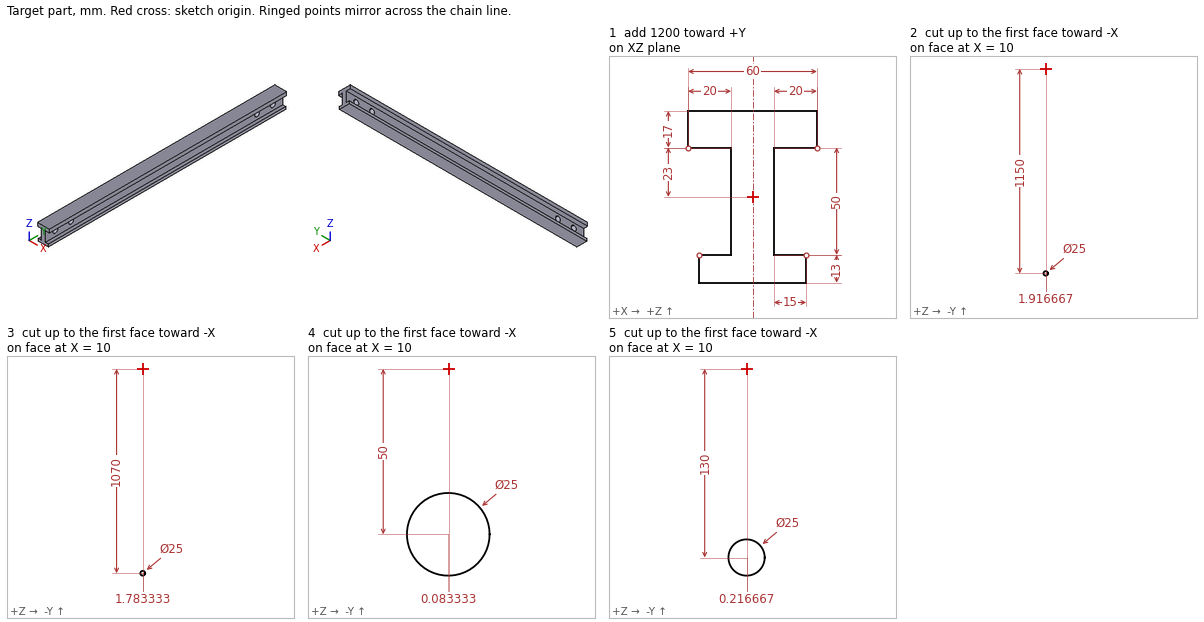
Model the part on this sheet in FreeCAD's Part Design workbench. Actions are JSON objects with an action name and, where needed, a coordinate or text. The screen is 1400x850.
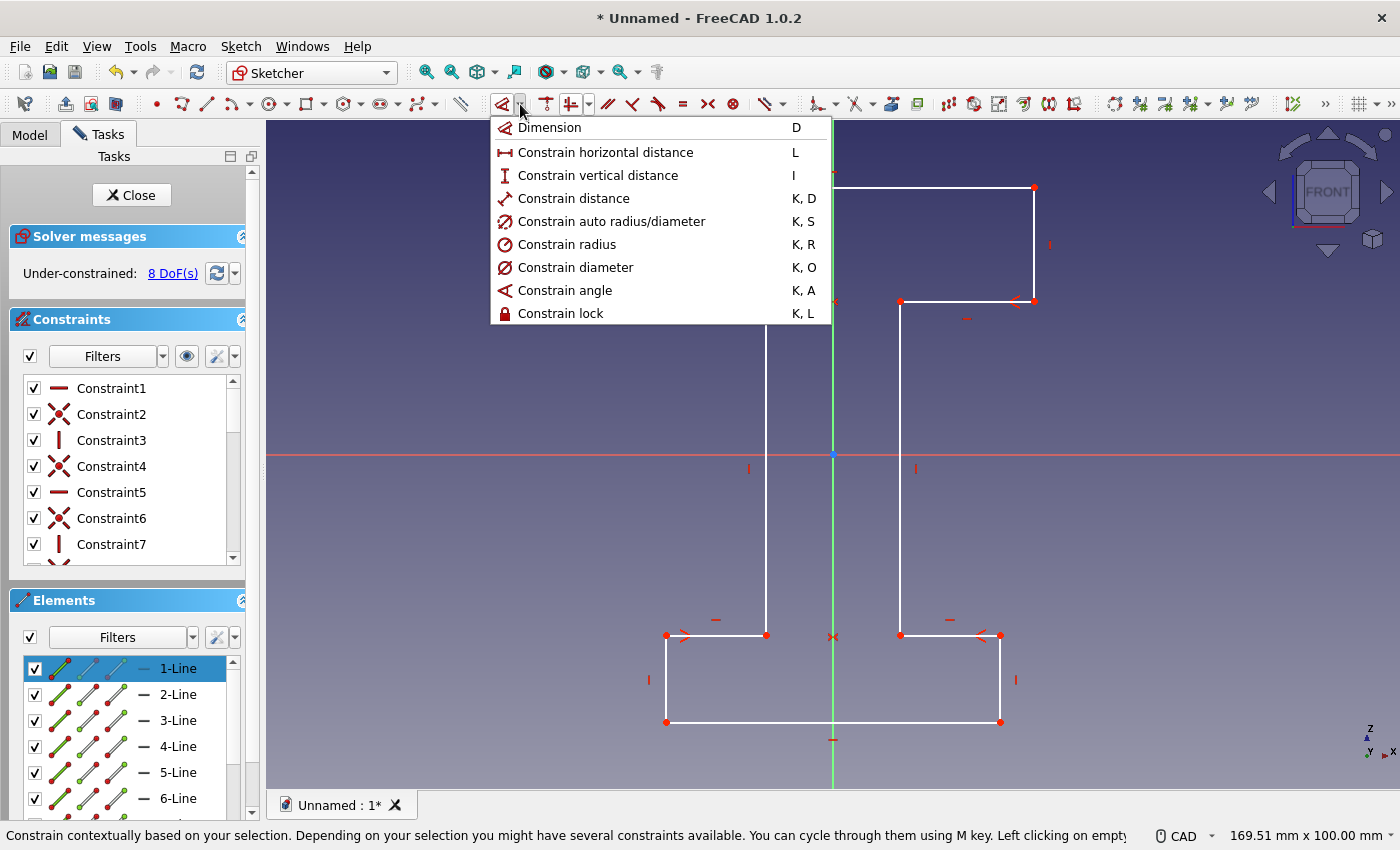
{"action": "left_click", "coordinate": [661, 152]}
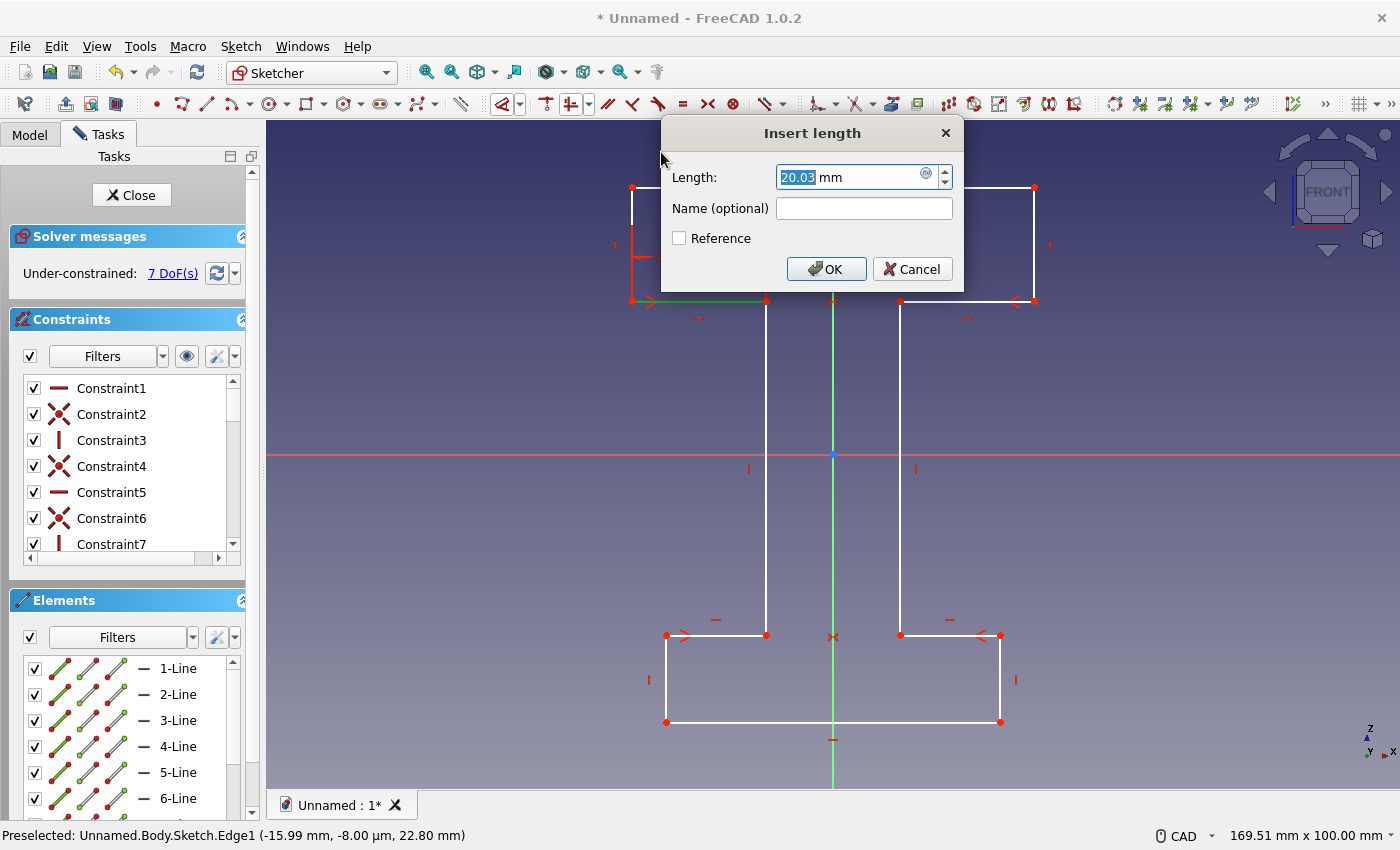
{"action": "type", "text": "20"}
{"action": "key", "text": "Return"}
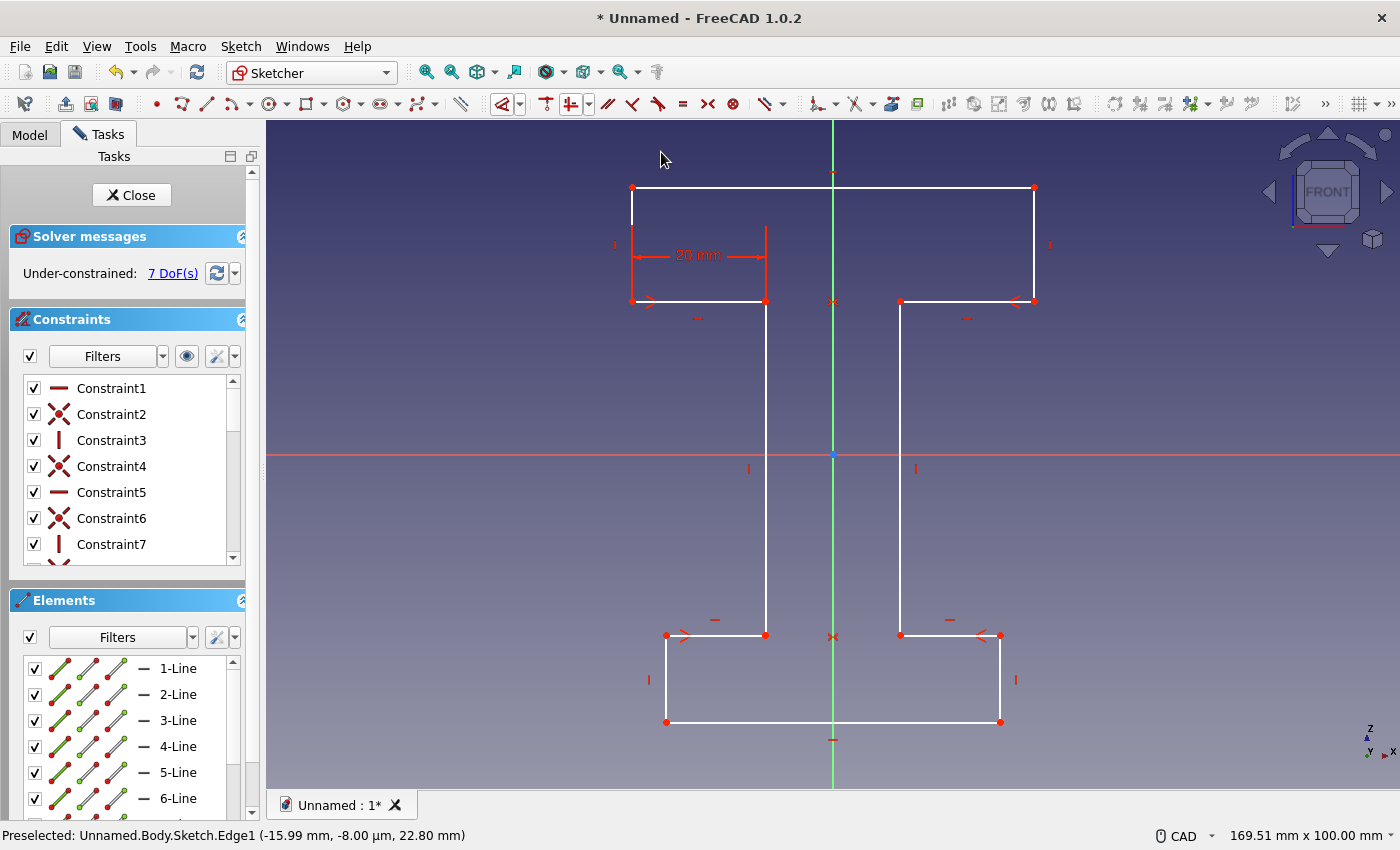
{"action": "left_click", "coordinate": [632, 268]}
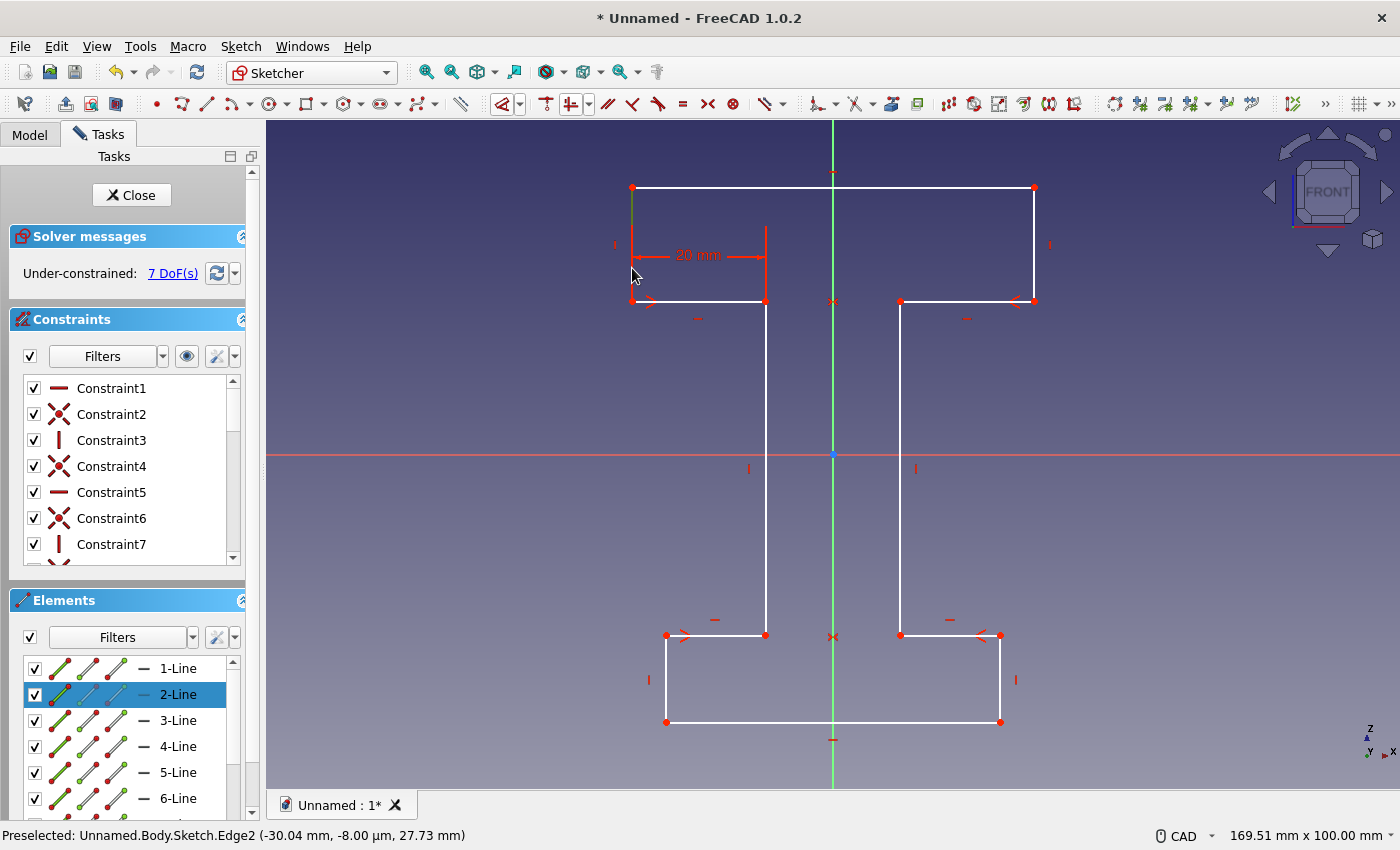
{"action": "left_click", "coordinate": [520, 104]}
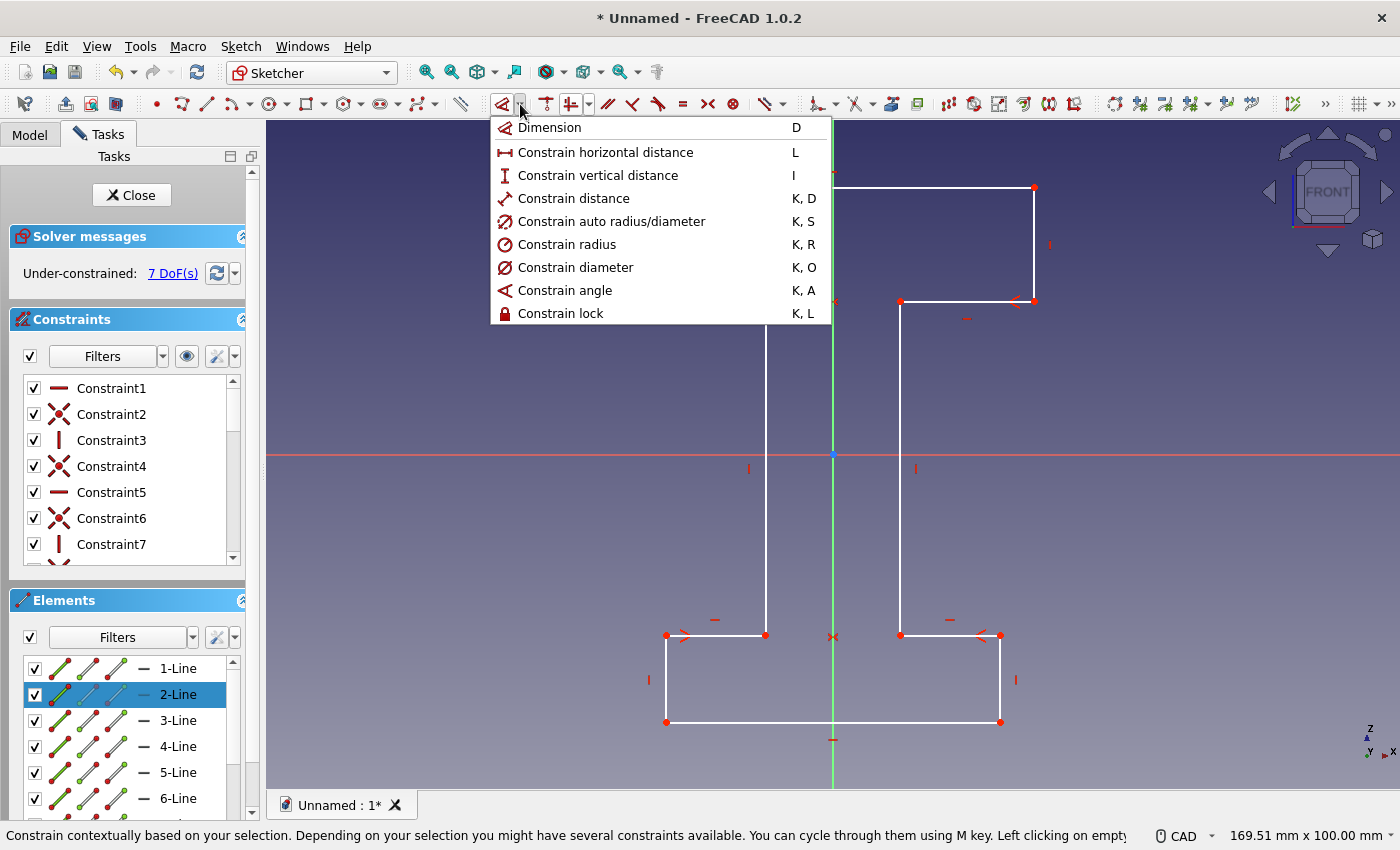
{"action": "left_click", "coordinate": [661, 176]}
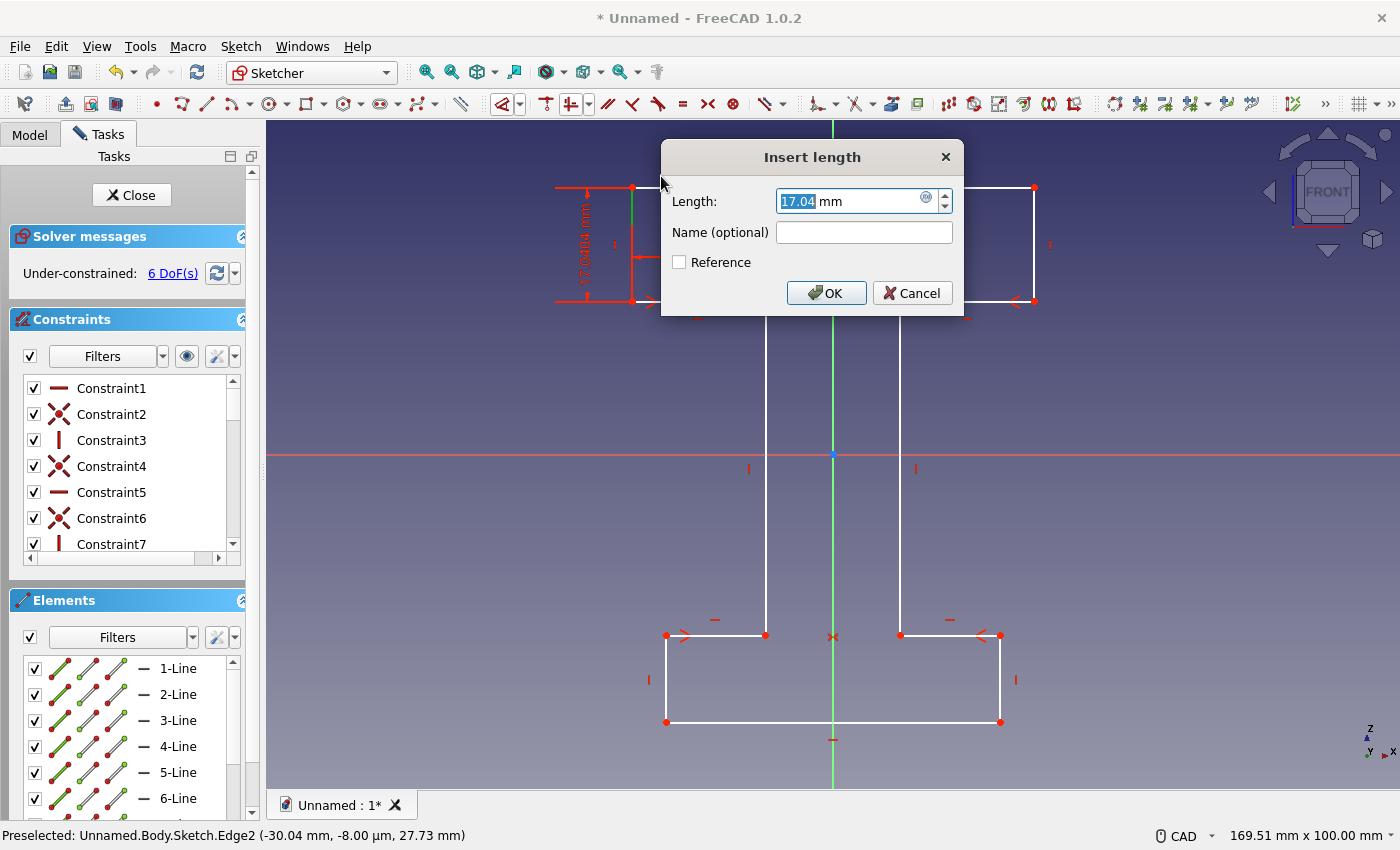
{"action": "type", "text": "17"}
{"action": "key", "text": "Return"}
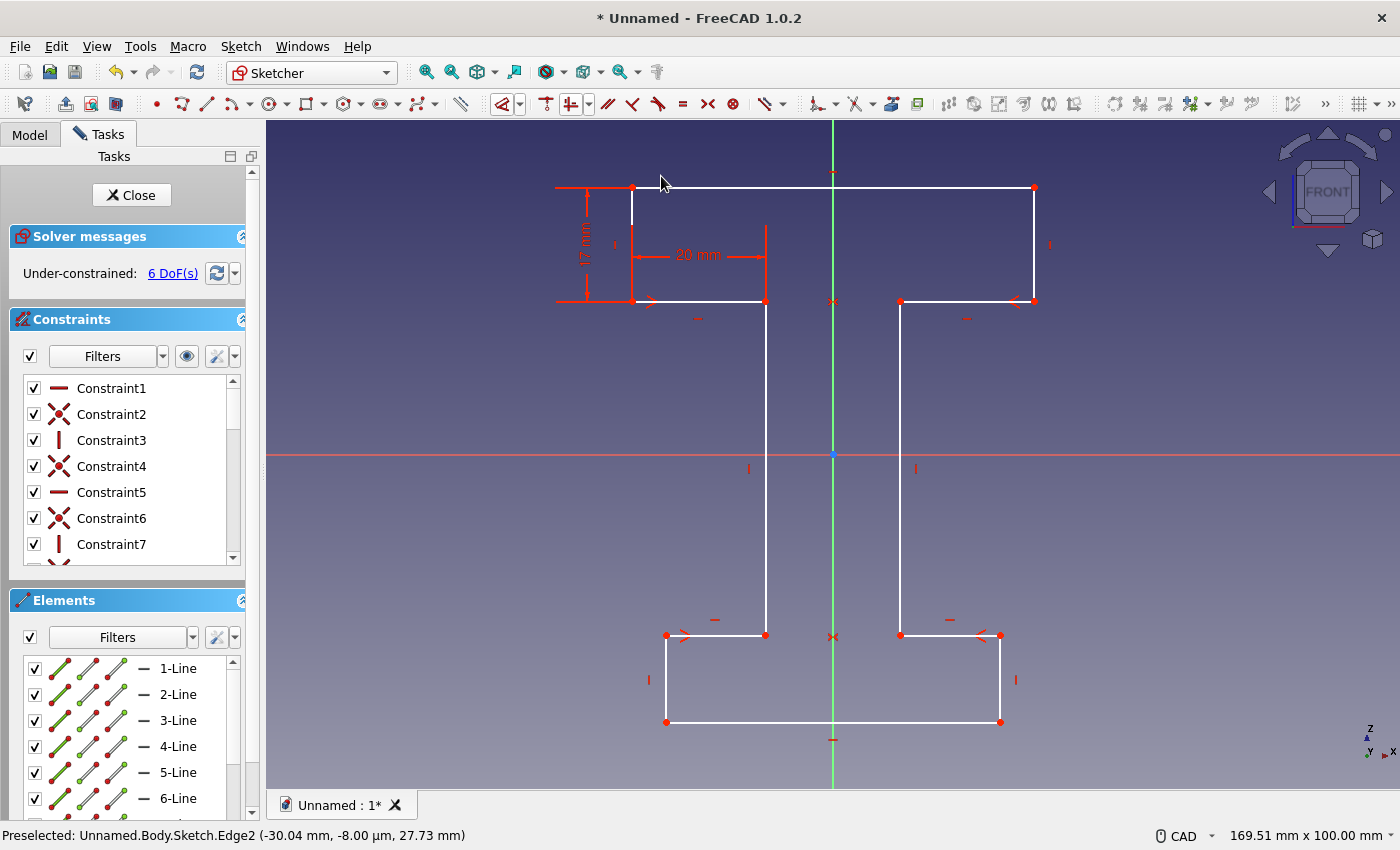
{"action": "left_click", "coordinate": [753, 188]}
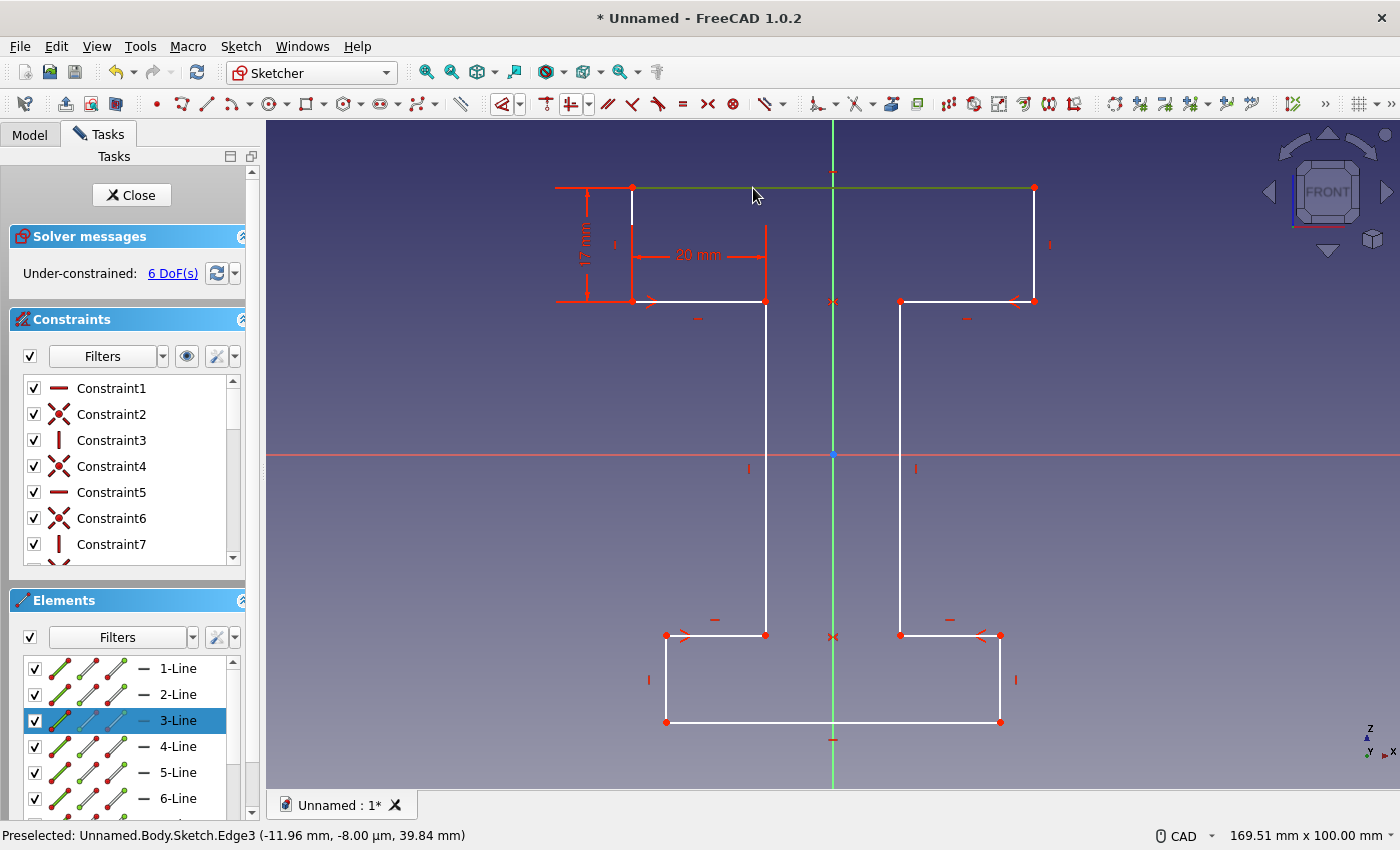
{"action": "left_click", "coordinate": [520, 104]}